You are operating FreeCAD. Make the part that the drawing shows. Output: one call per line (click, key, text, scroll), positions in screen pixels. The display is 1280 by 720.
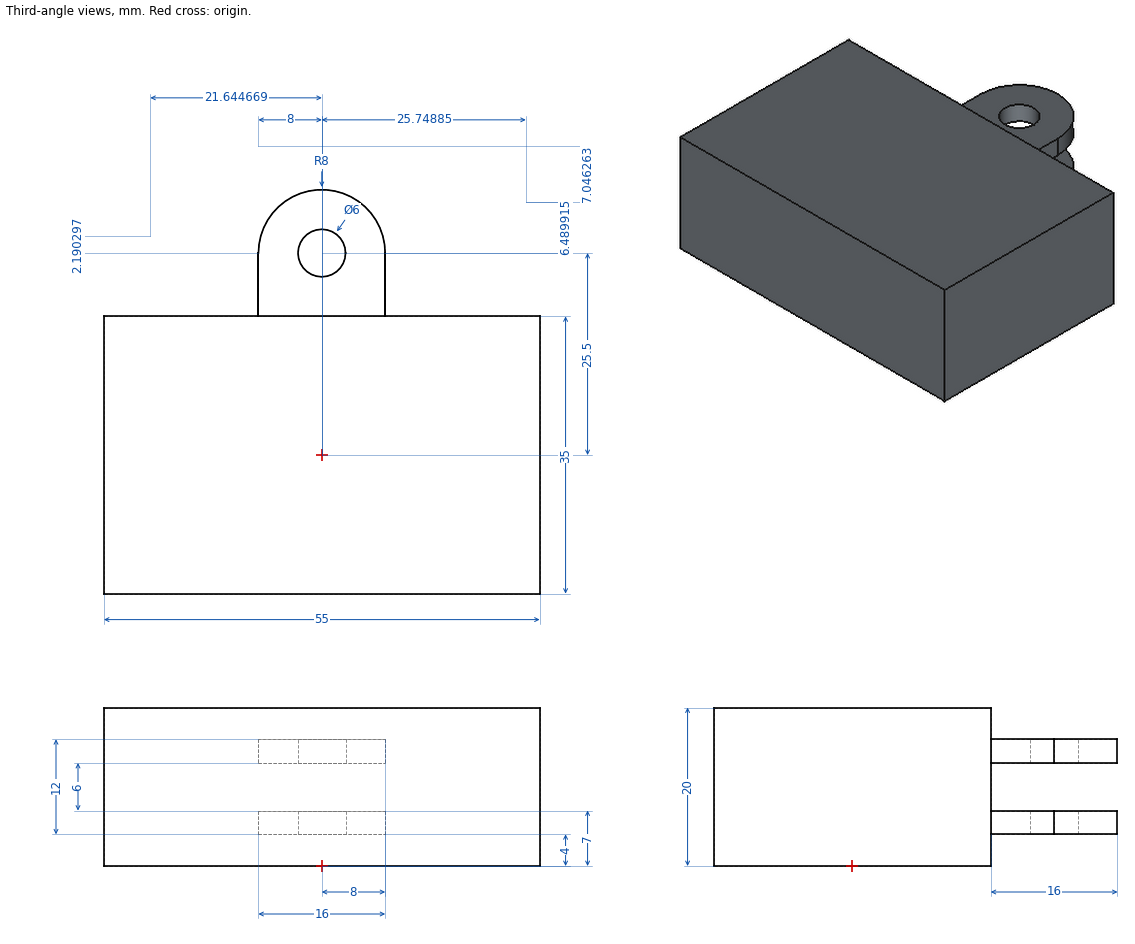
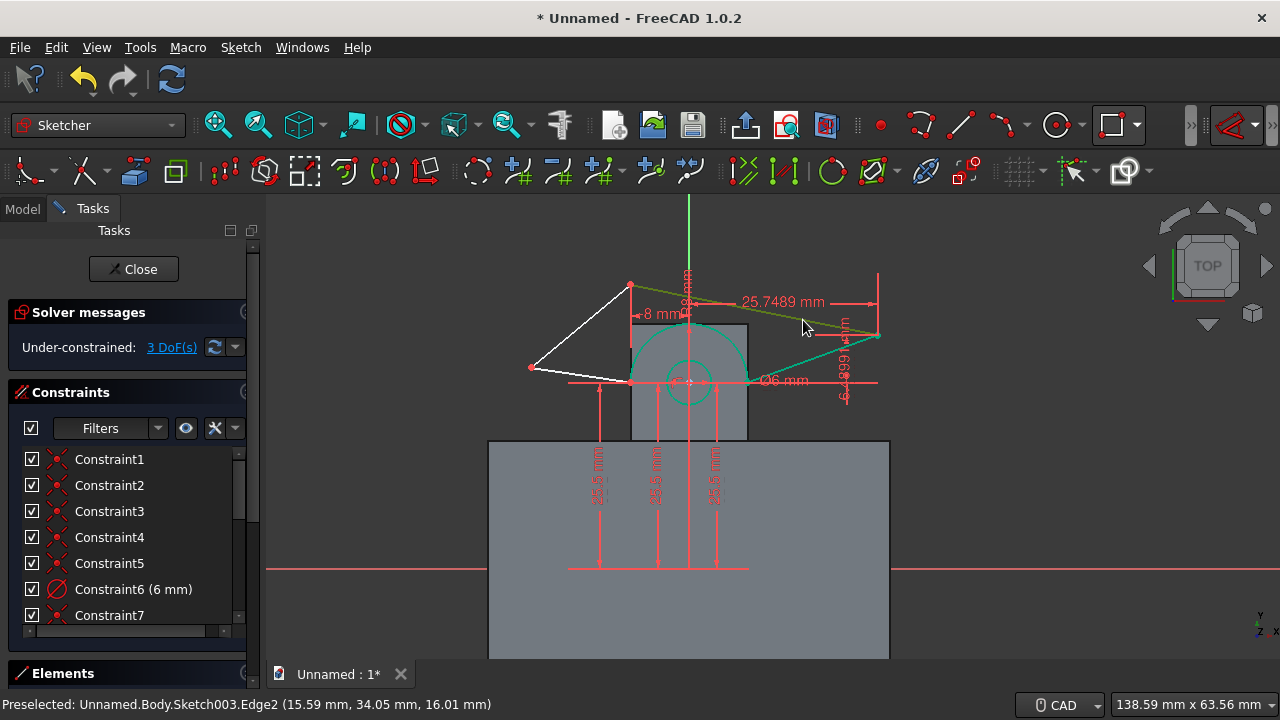
click(1258, 126)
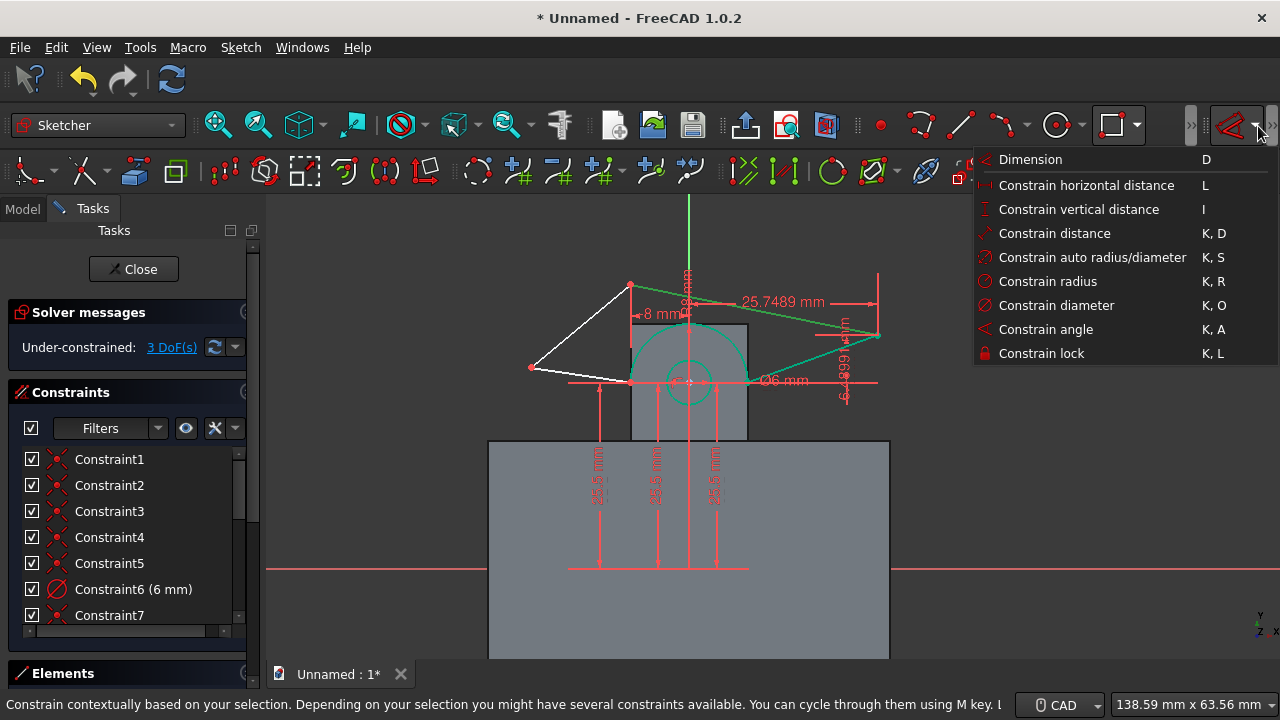
click(1126, 209)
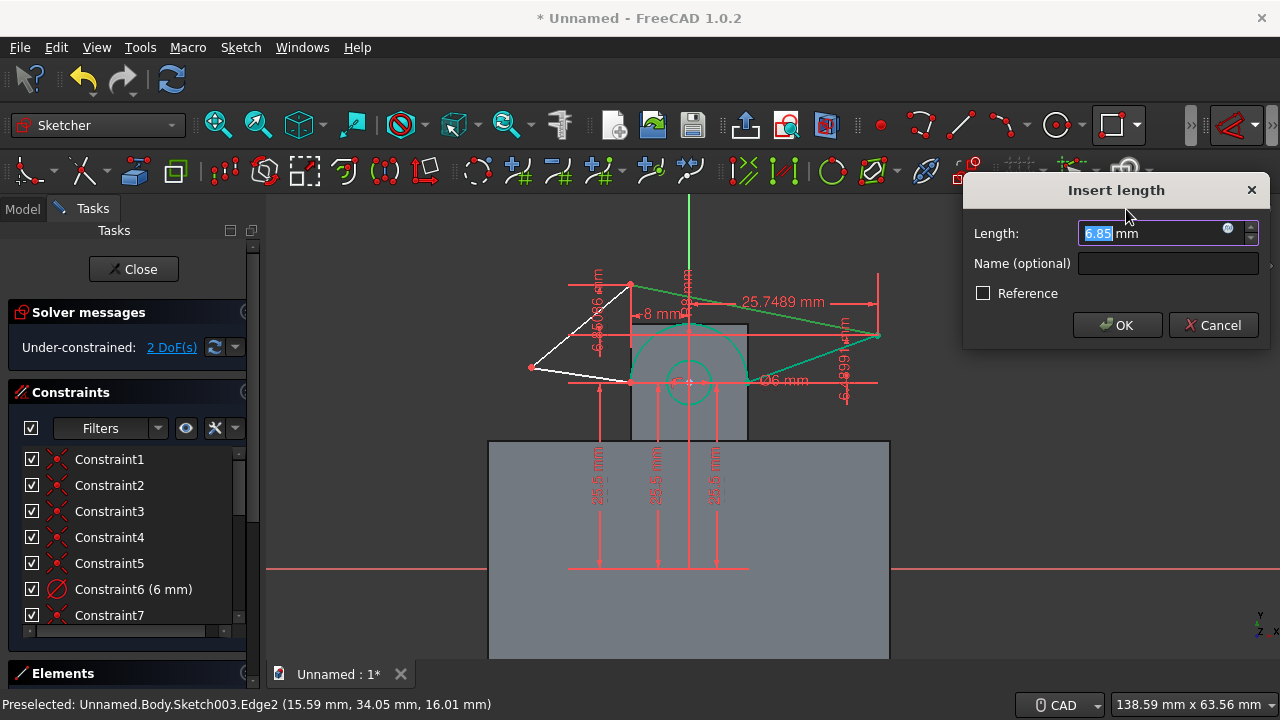
text(7.046263)
key(Return)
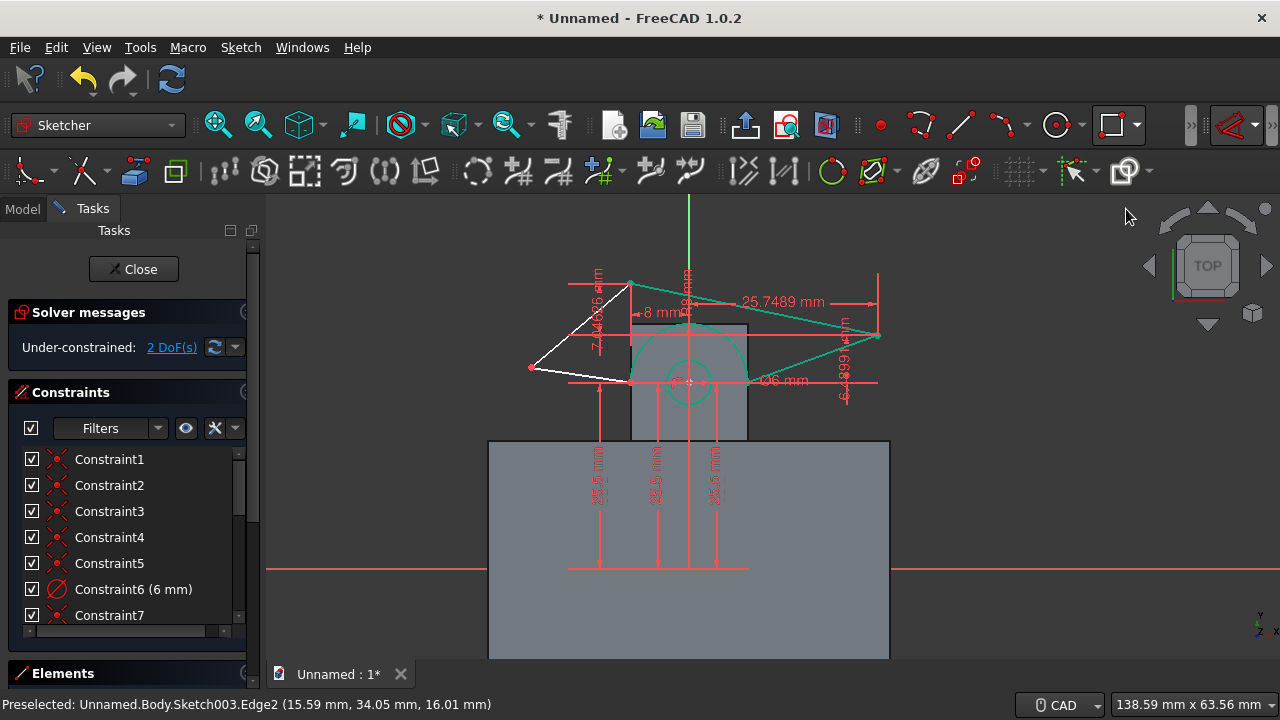
scroll(561, 372, up, 5)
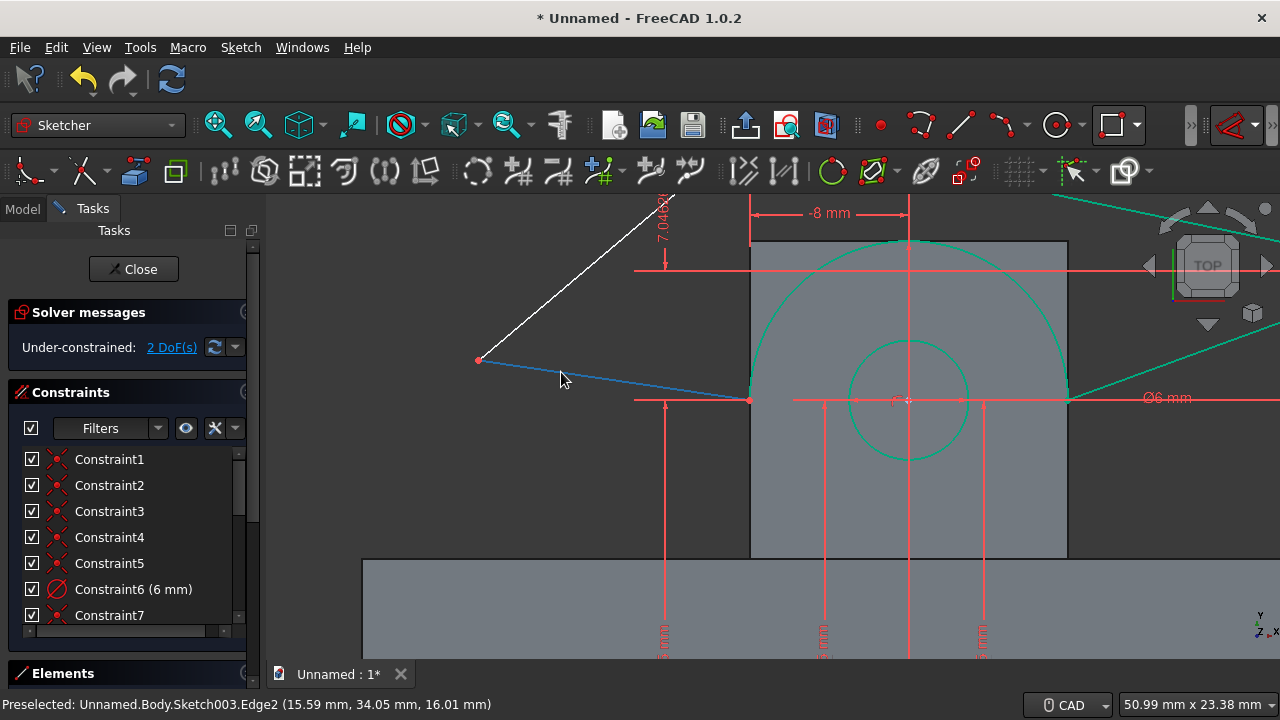
click(560, 372)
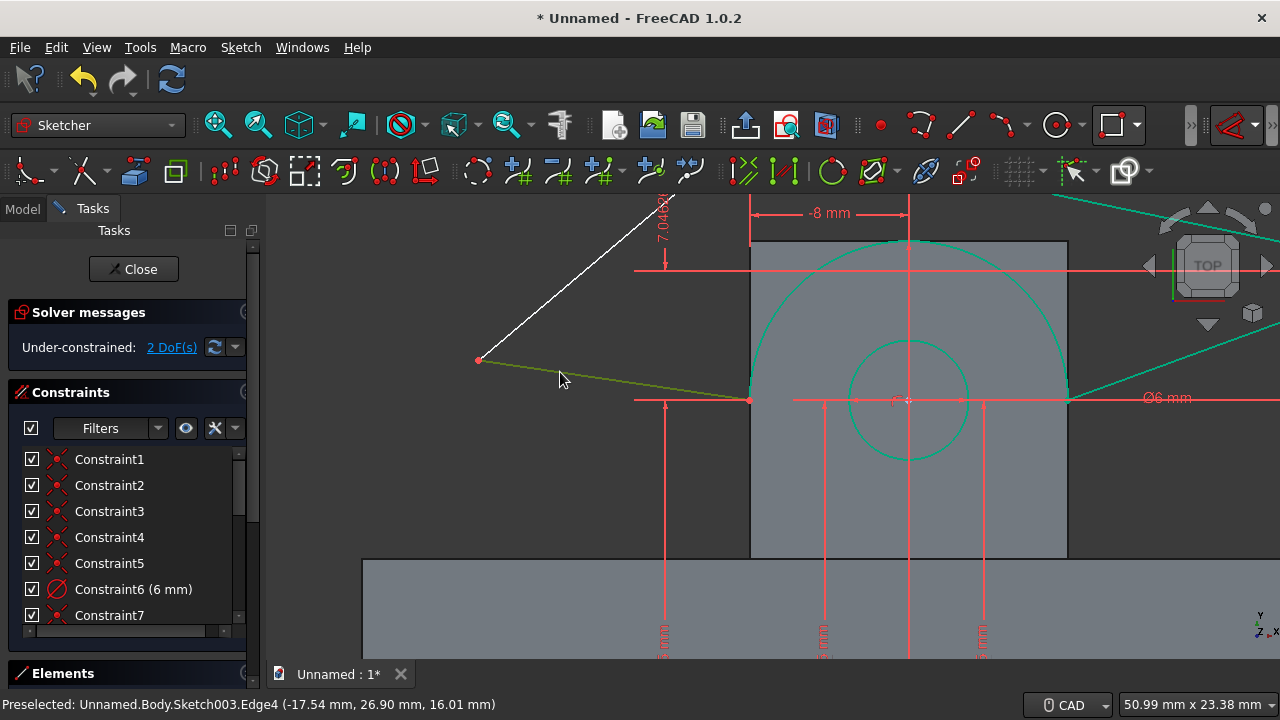
click(1258, 126)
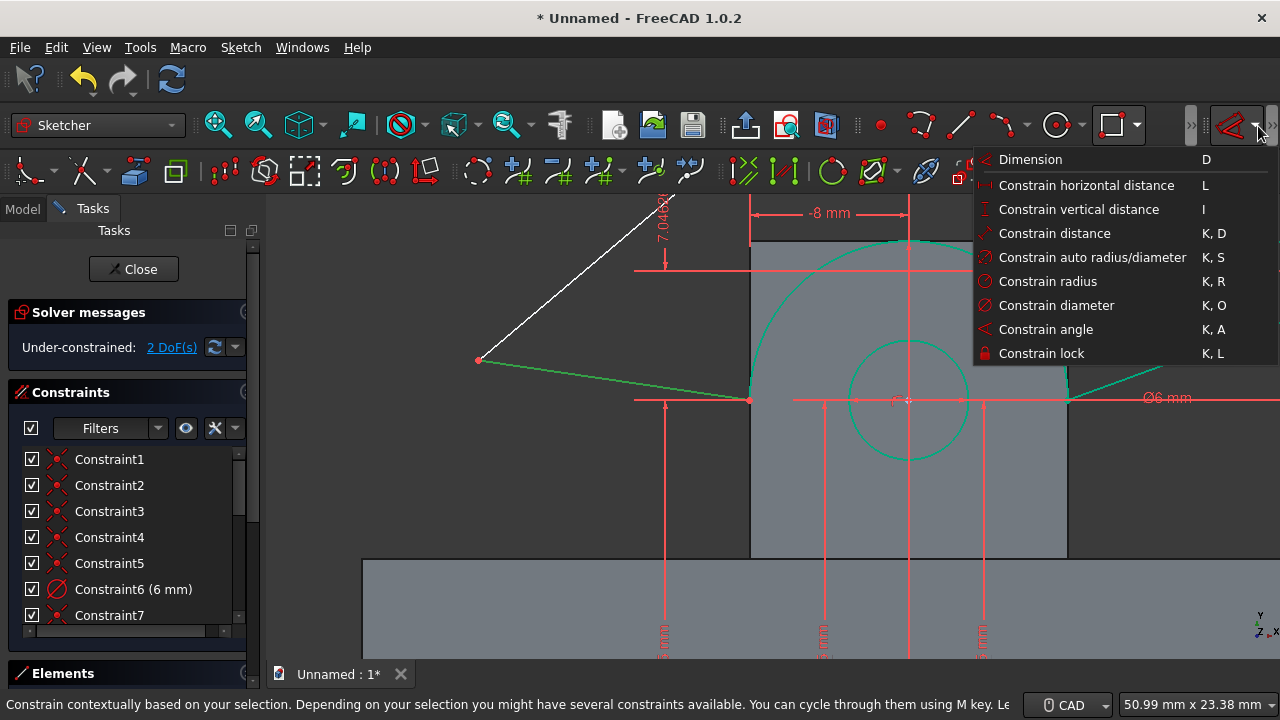
click(1126, 209)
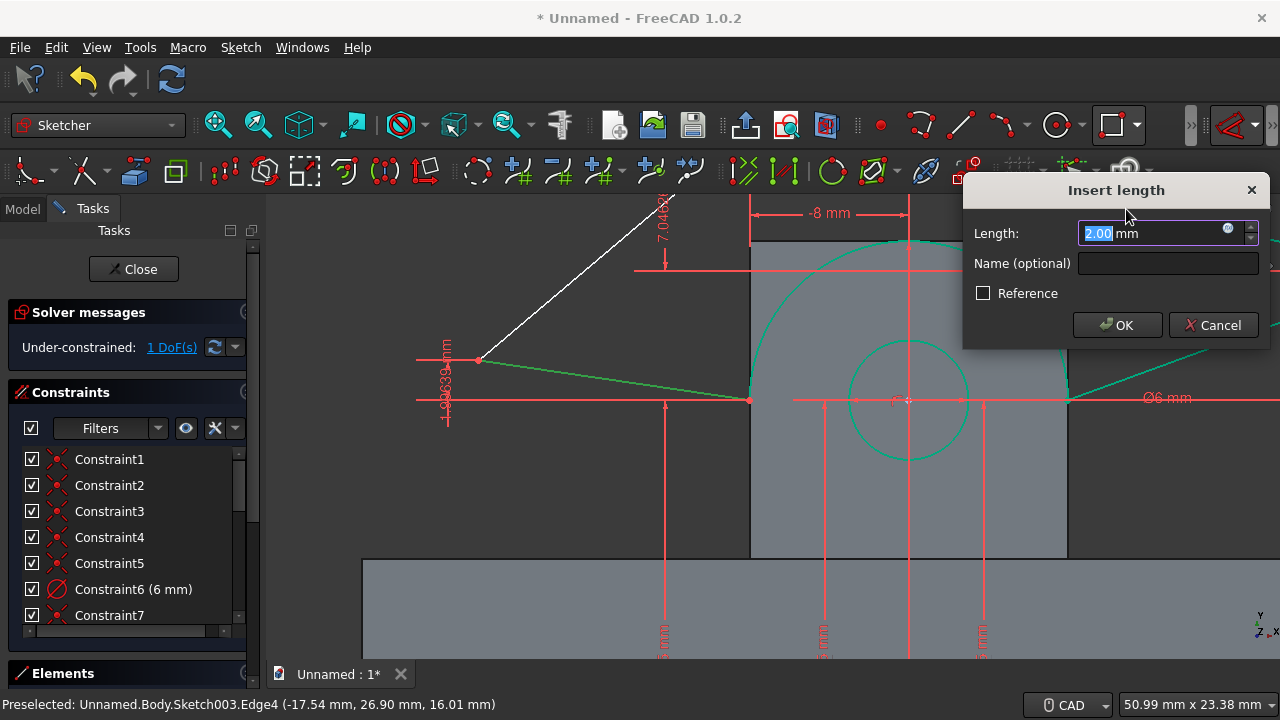
text(2.190297)
key(Return)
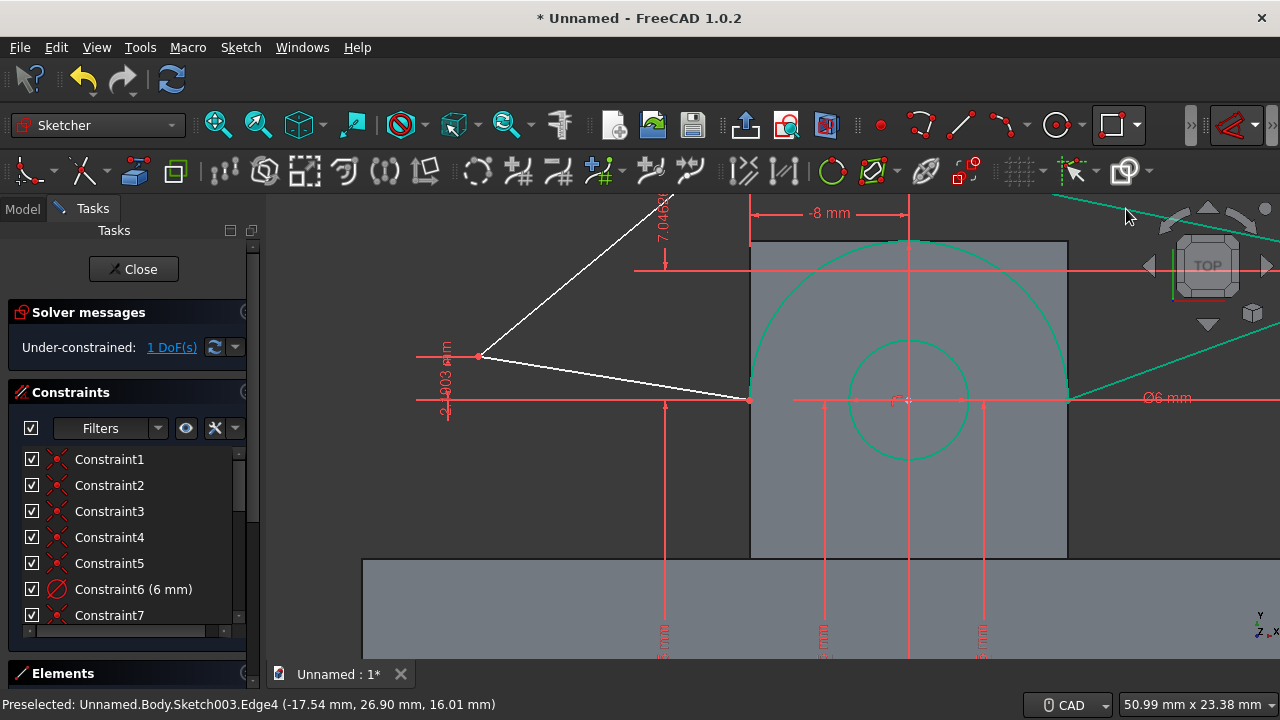
click(479, 357)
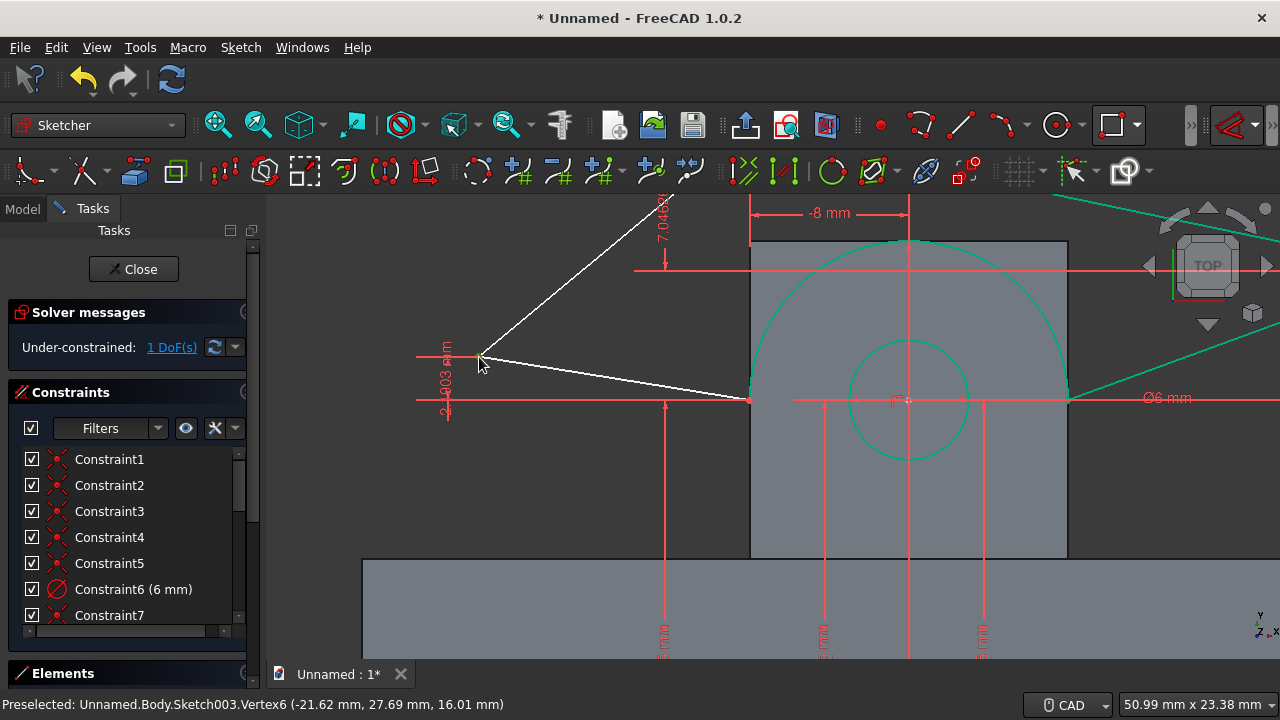
key(l)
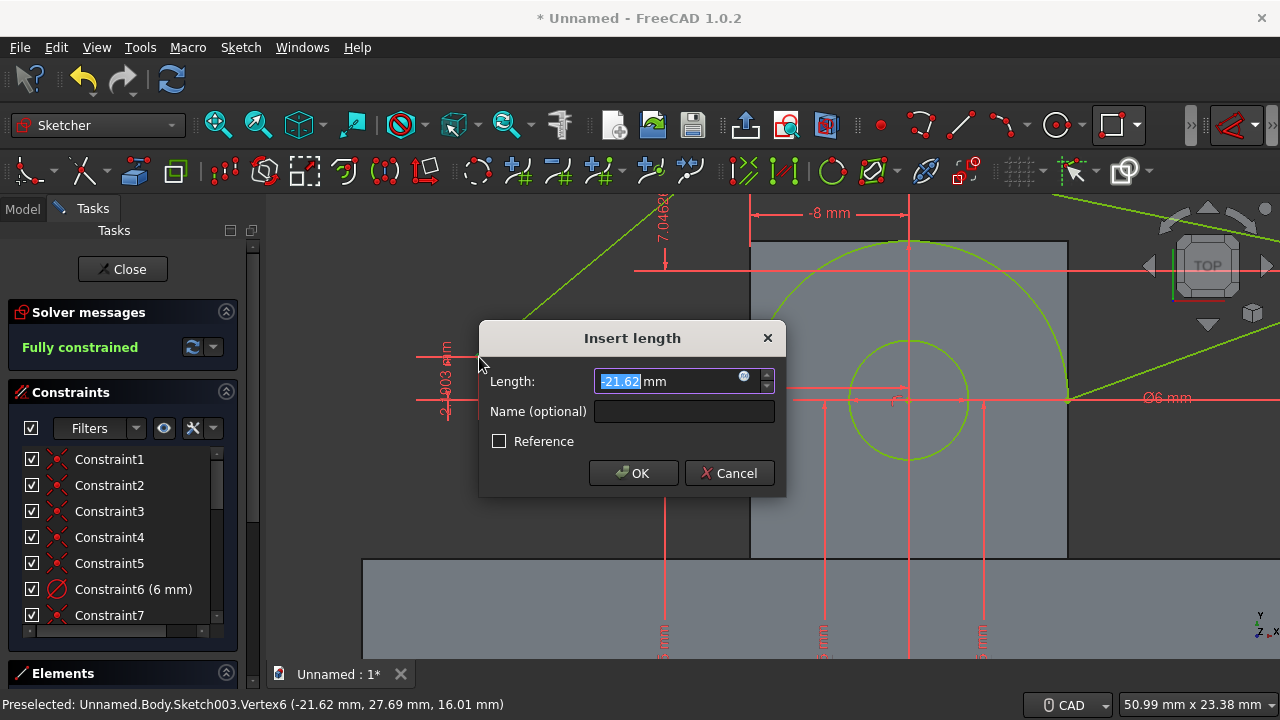
text(-21.644669)
key(Return)